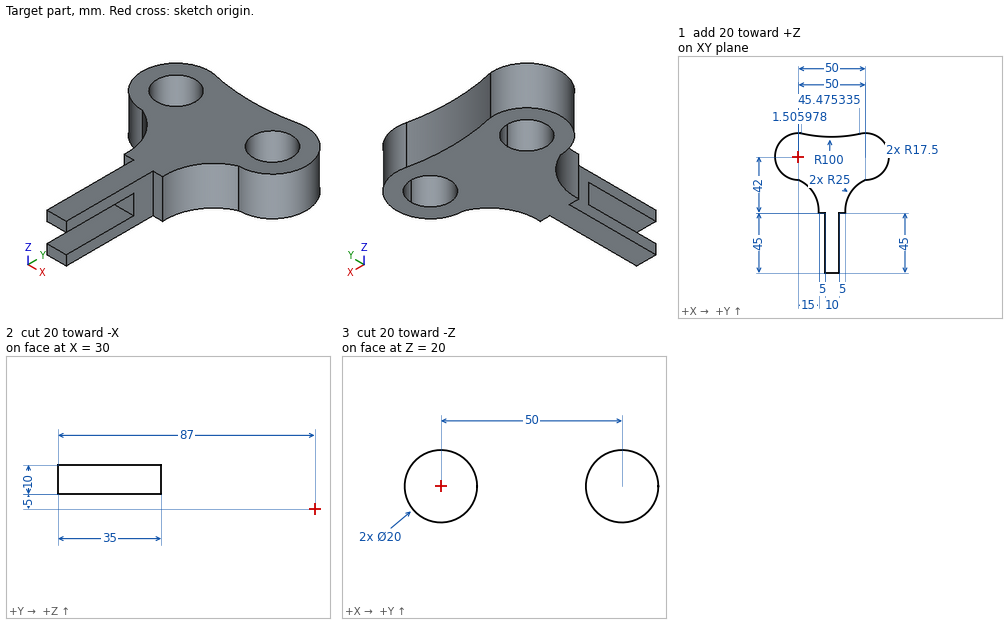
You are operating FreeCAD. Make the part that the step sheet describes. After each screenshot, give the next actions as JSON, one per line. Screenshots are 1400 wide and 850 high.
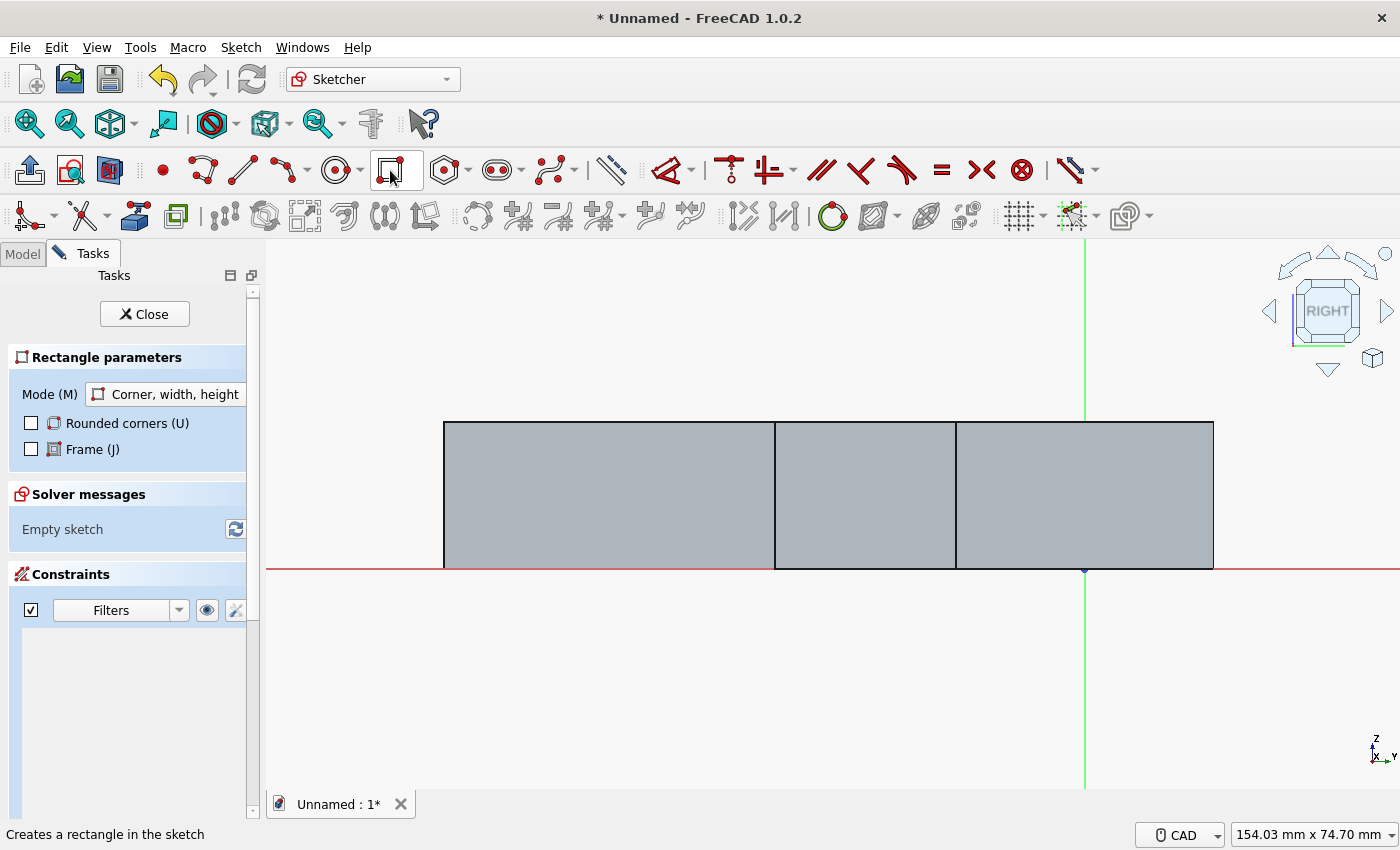
{"action": "left_click", "coordinate": [444, 459]}
{"action": "left_click", "coordinate": [702, 532]}
{"action": "key", "text": "Escape"}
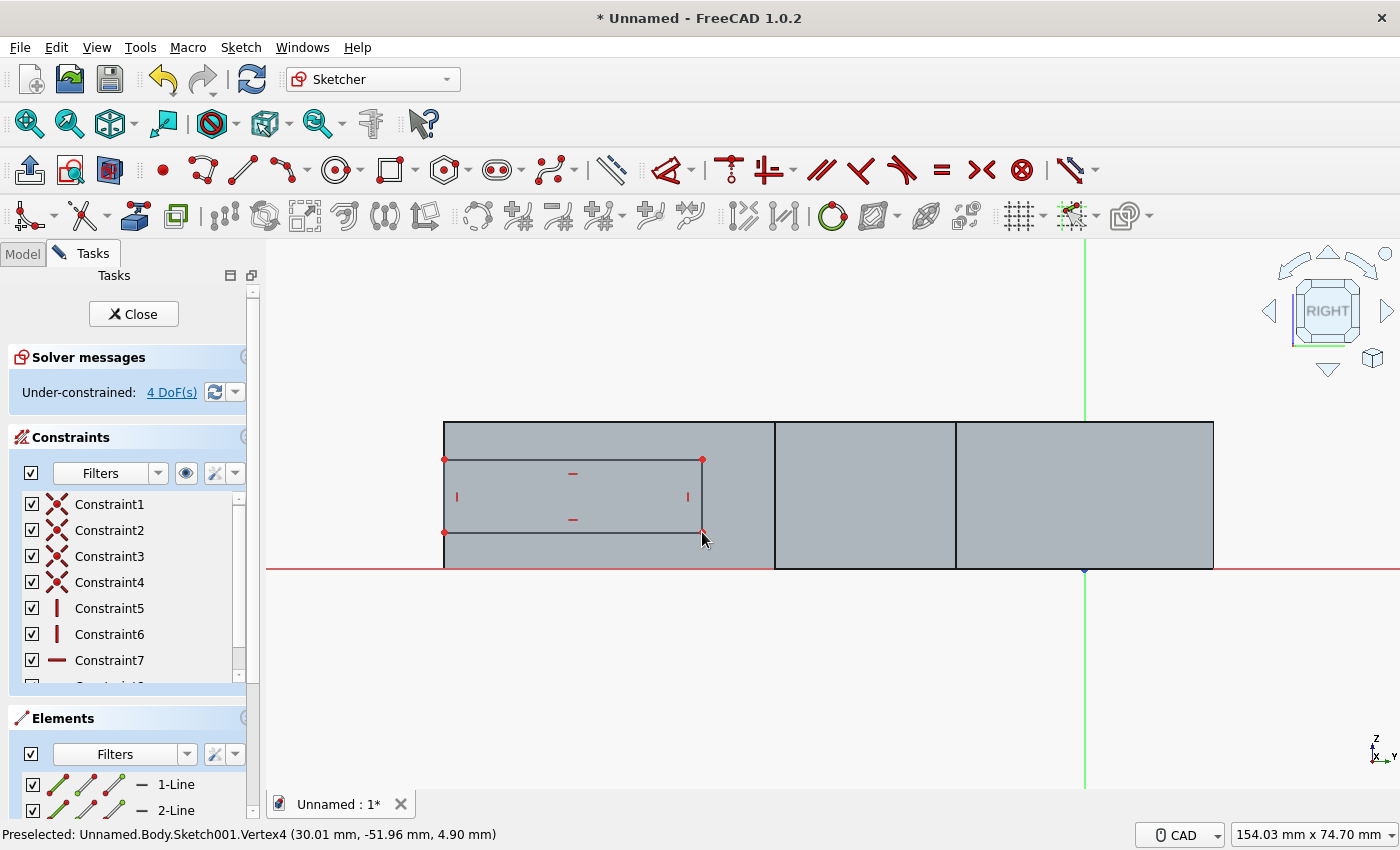
{"action": "left_click", "coordinate": [666, 170]}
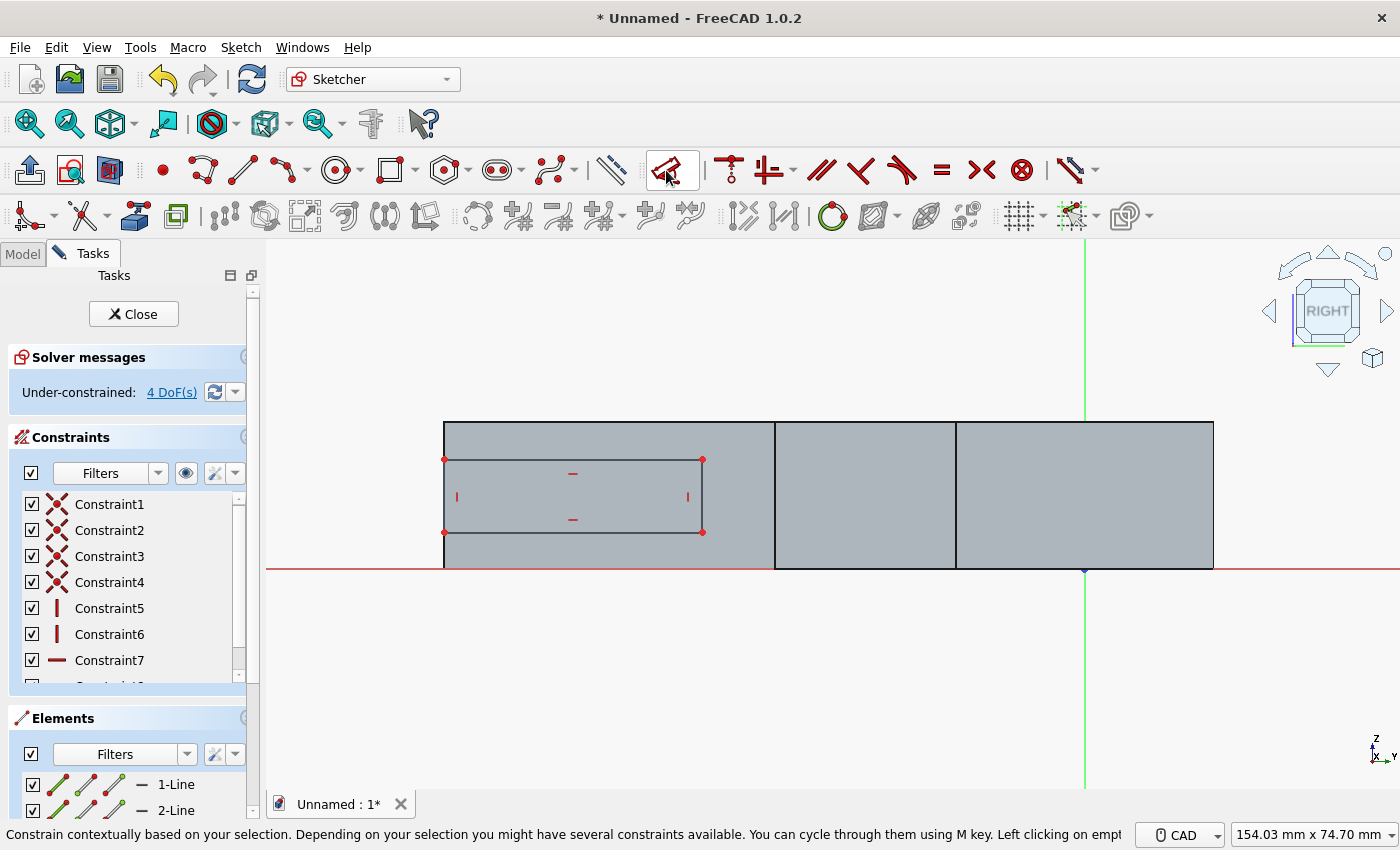
{"action": "left_click", "coordinate": [444, 482]}
{"action": "left_click", "coordinate": [410, 496]}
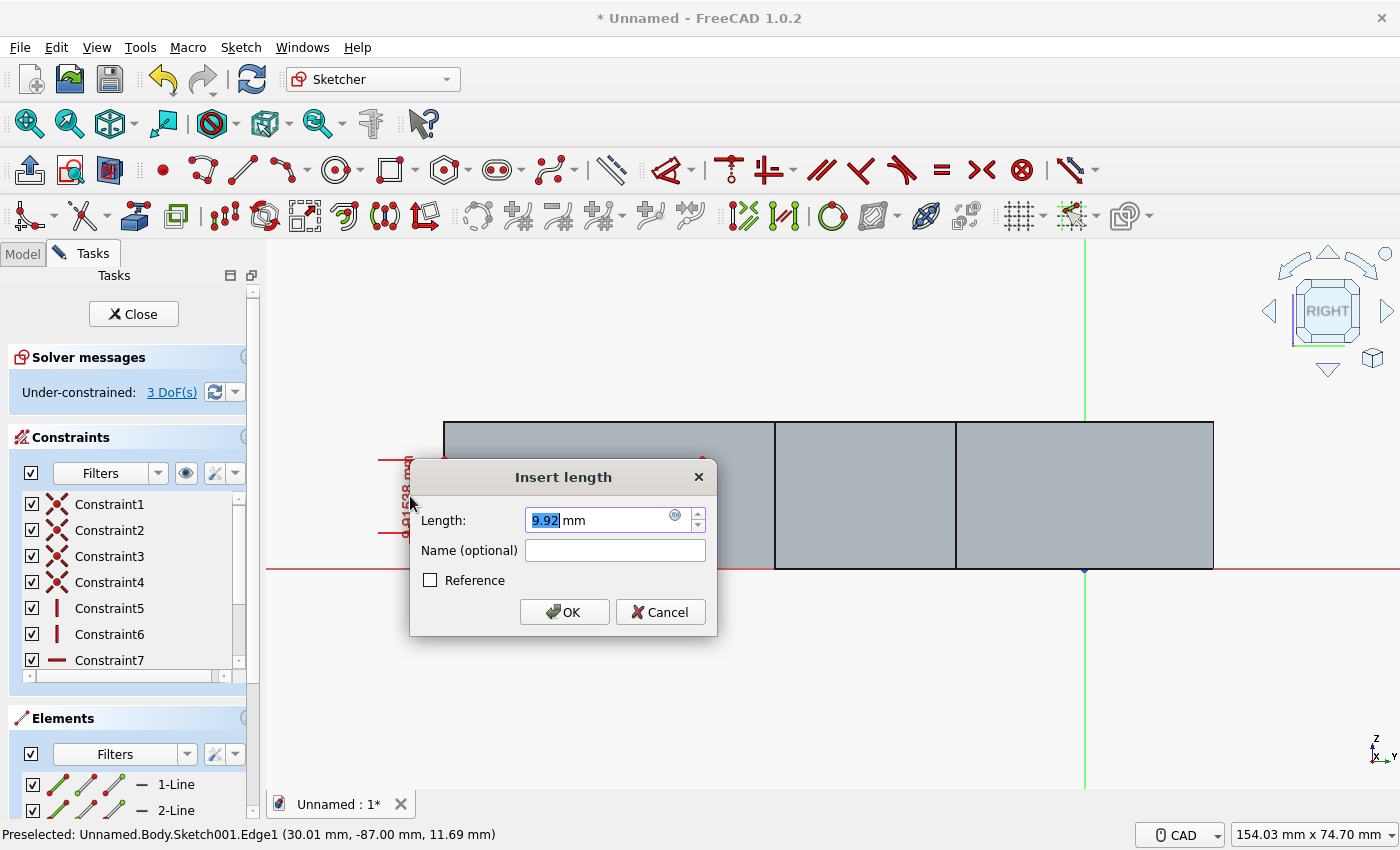
{"action": "type", "text": "10"}
{"action": "key", "text": "Return"}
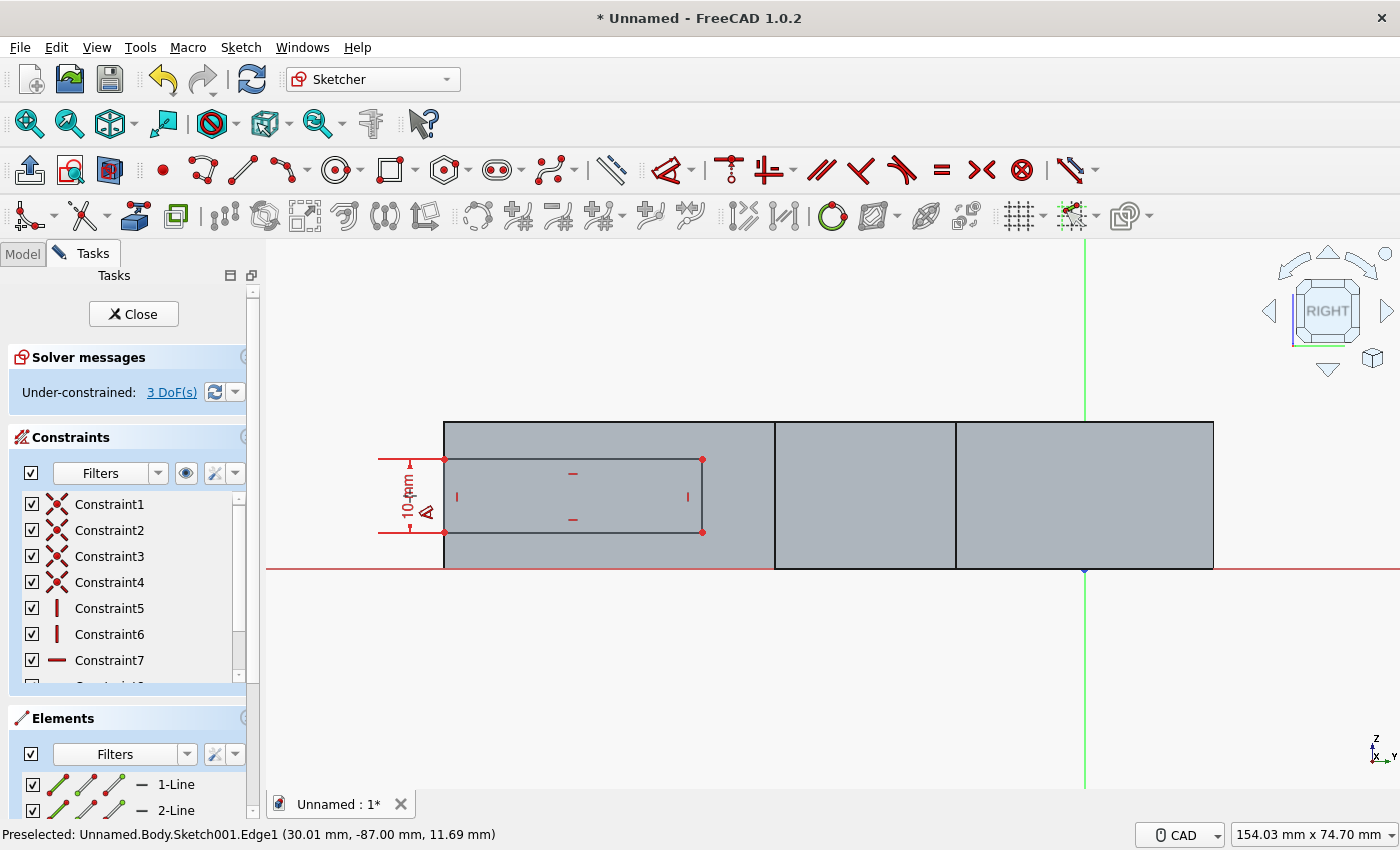
{"action": "left_click", "coordinate": [521, 533]}
{"action": "left_click", "coordinate": [573, 499]}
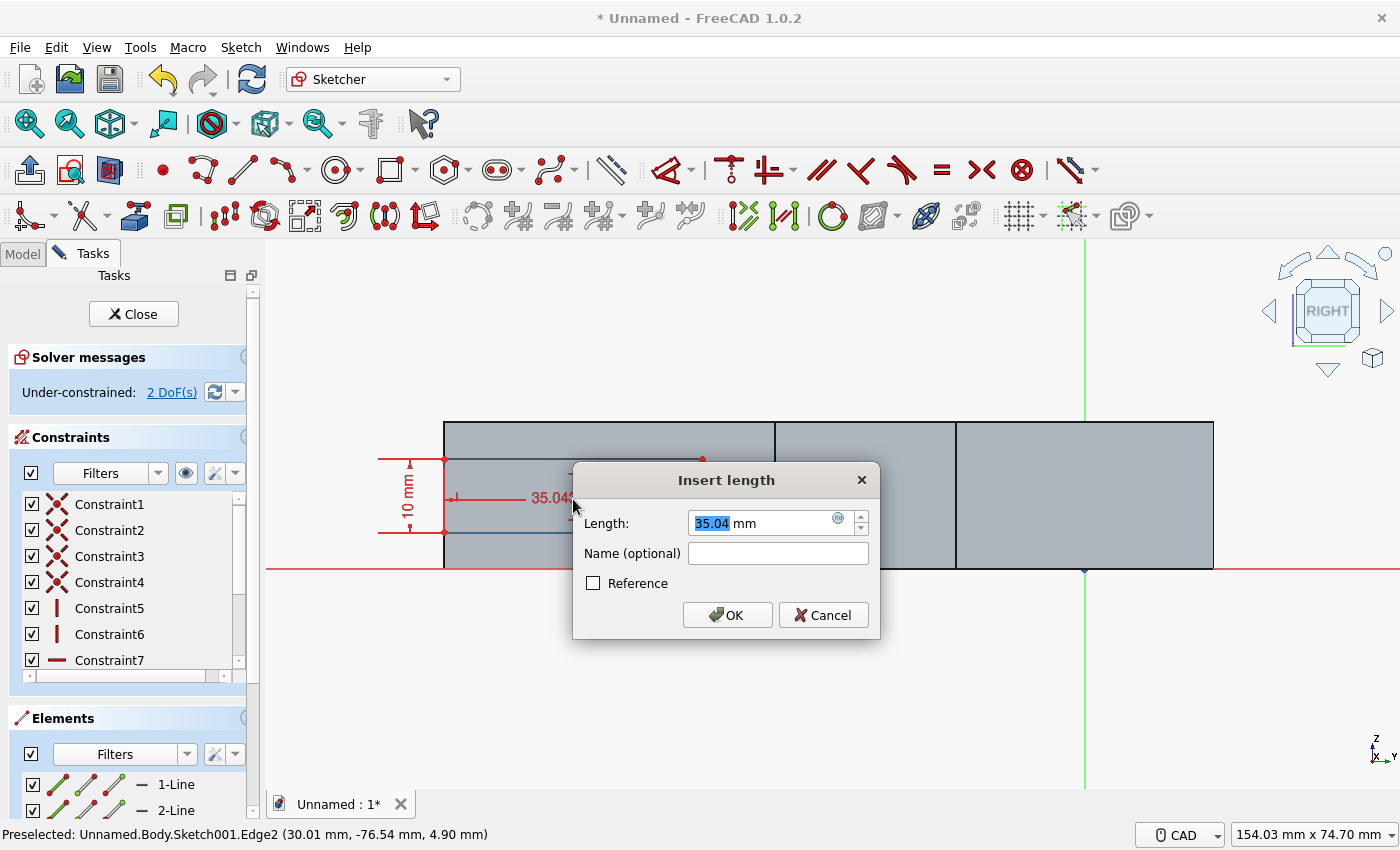
{"action": "type", "text": "35"}
{"action": "key", "text": "Return"}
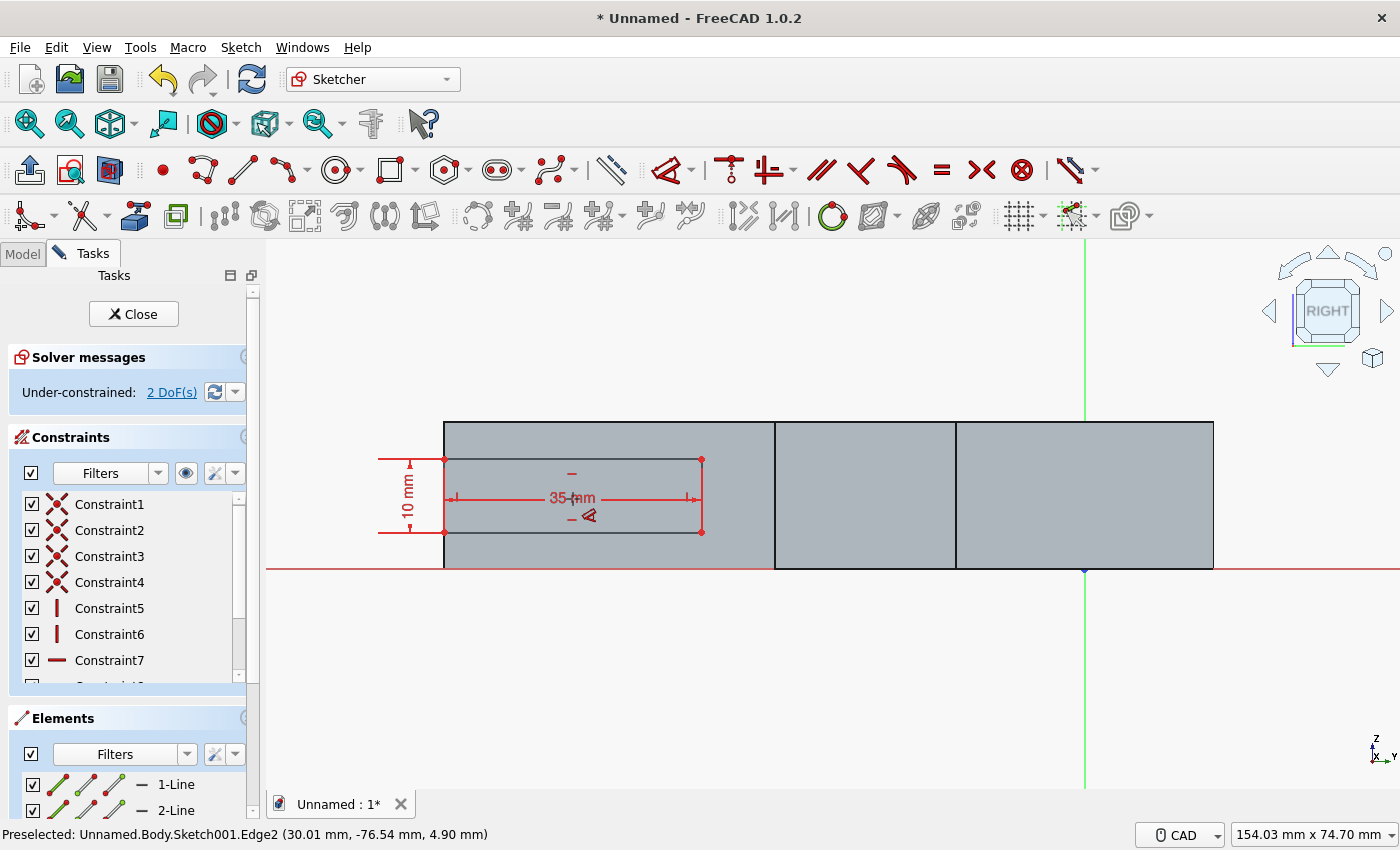
{"action": "left_click", "coordinate": [444, 533]}
{"action": "left_click", "coordinate": [1119, 551]}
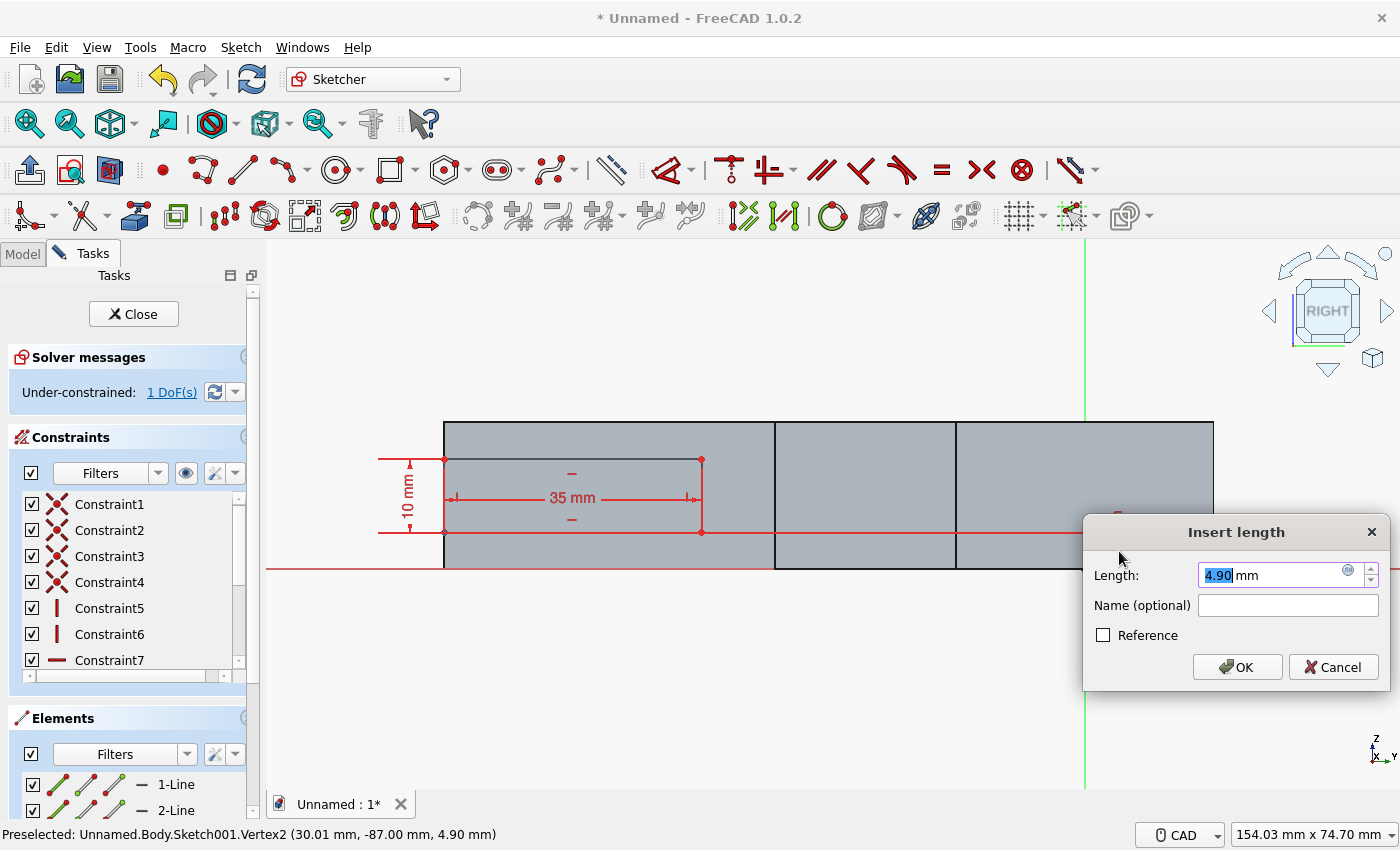
{"action": "type", "text": "5"}
{"action": "key", "text": "Return"}